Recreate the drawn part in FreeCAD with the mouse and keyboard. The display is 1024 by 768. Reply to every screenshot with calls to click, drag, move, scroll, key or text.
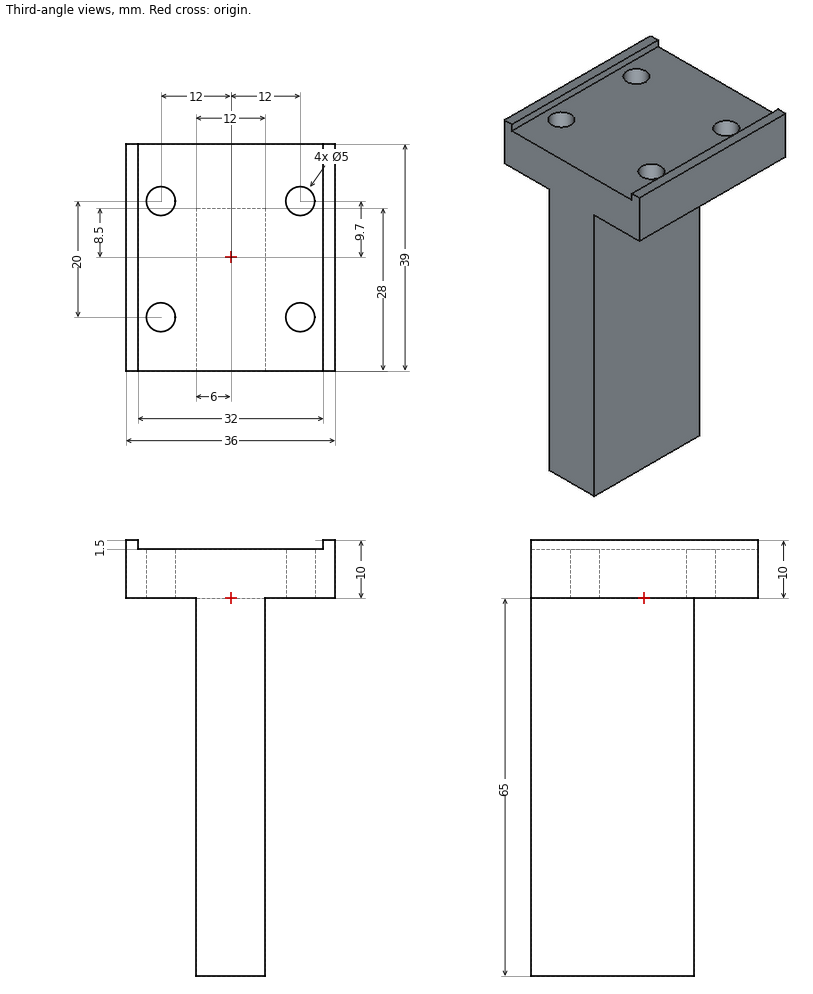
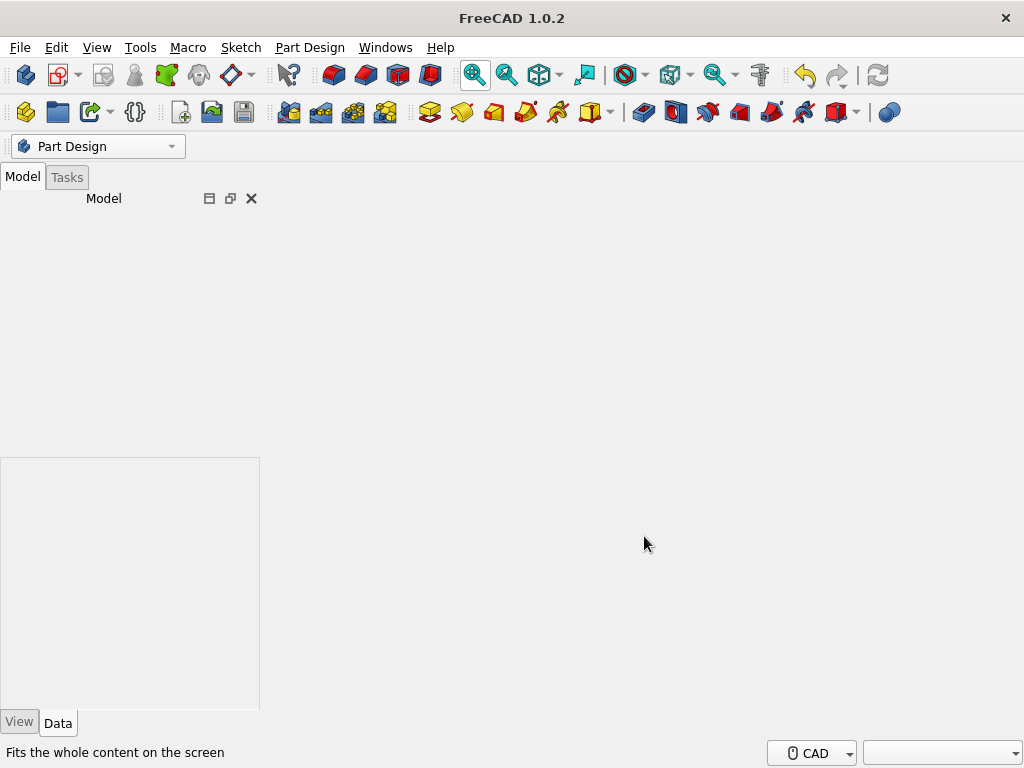
key(ctrl+n)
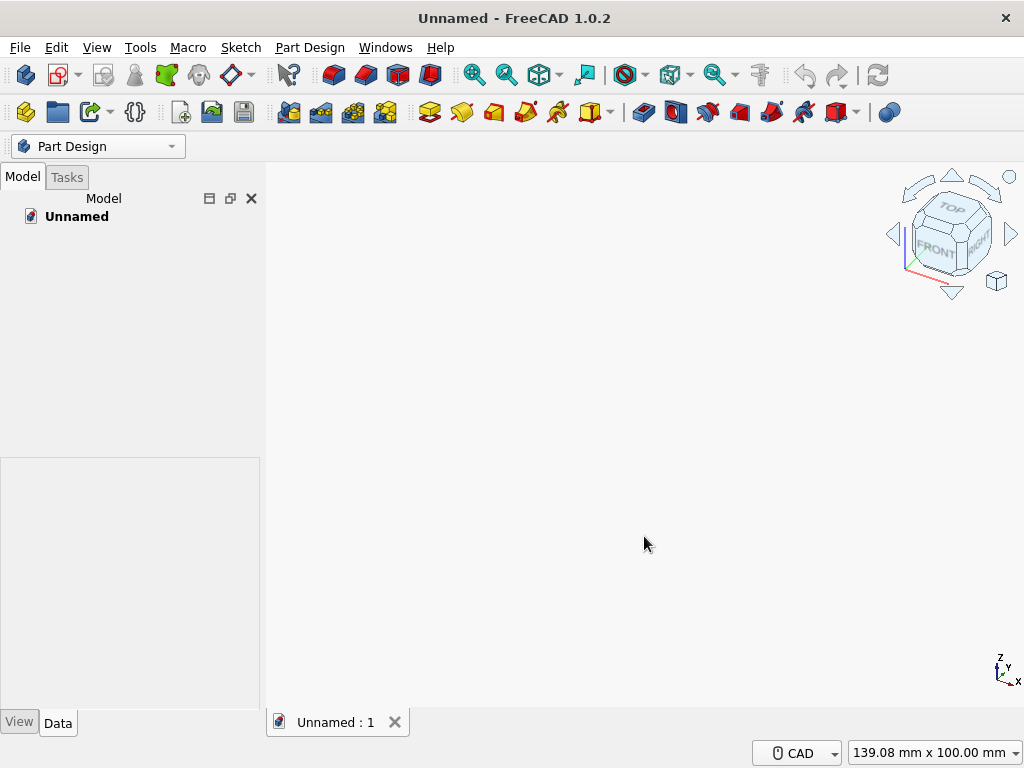
click(58, 76)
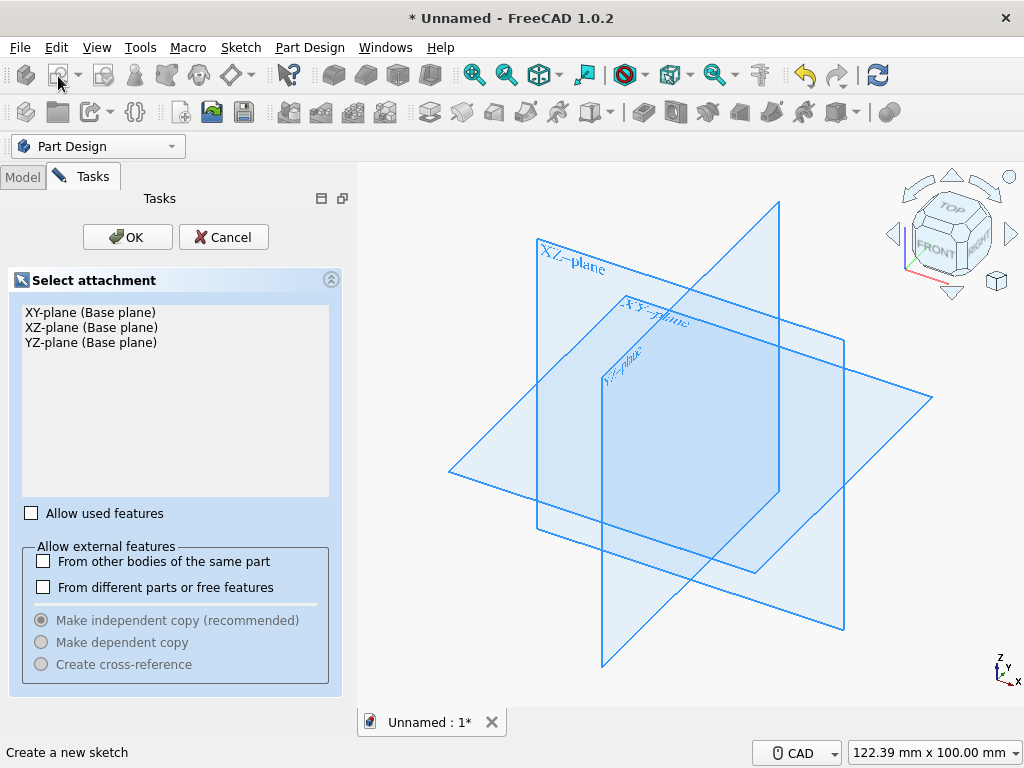
click(82, 312)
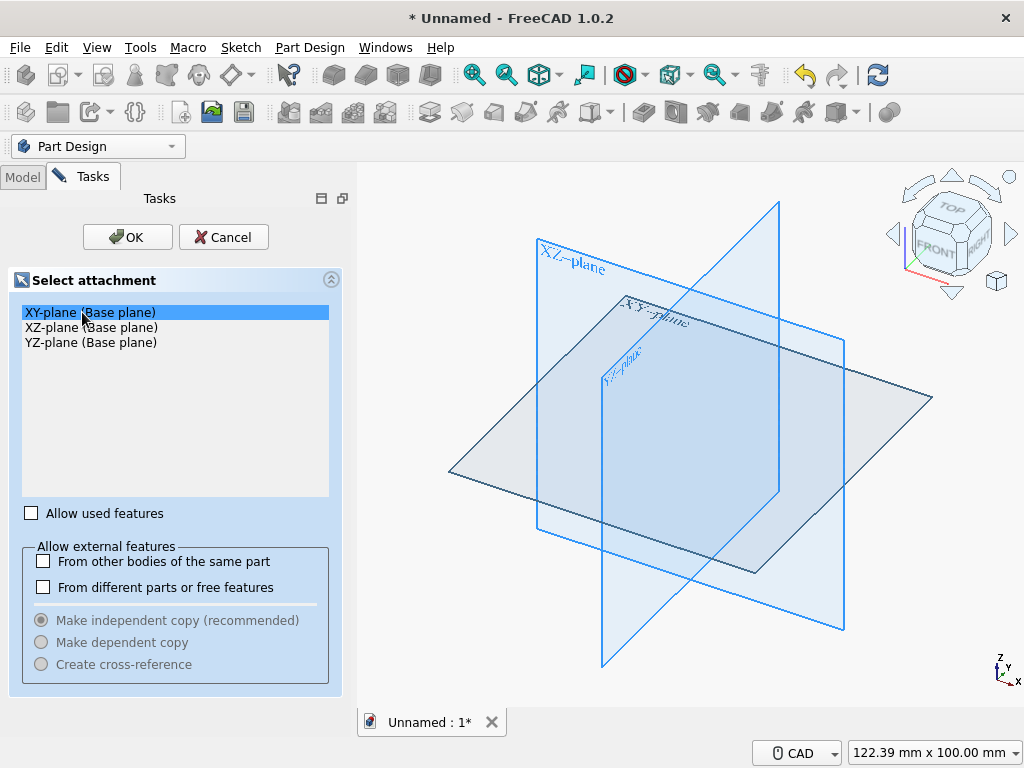
click(128, 237)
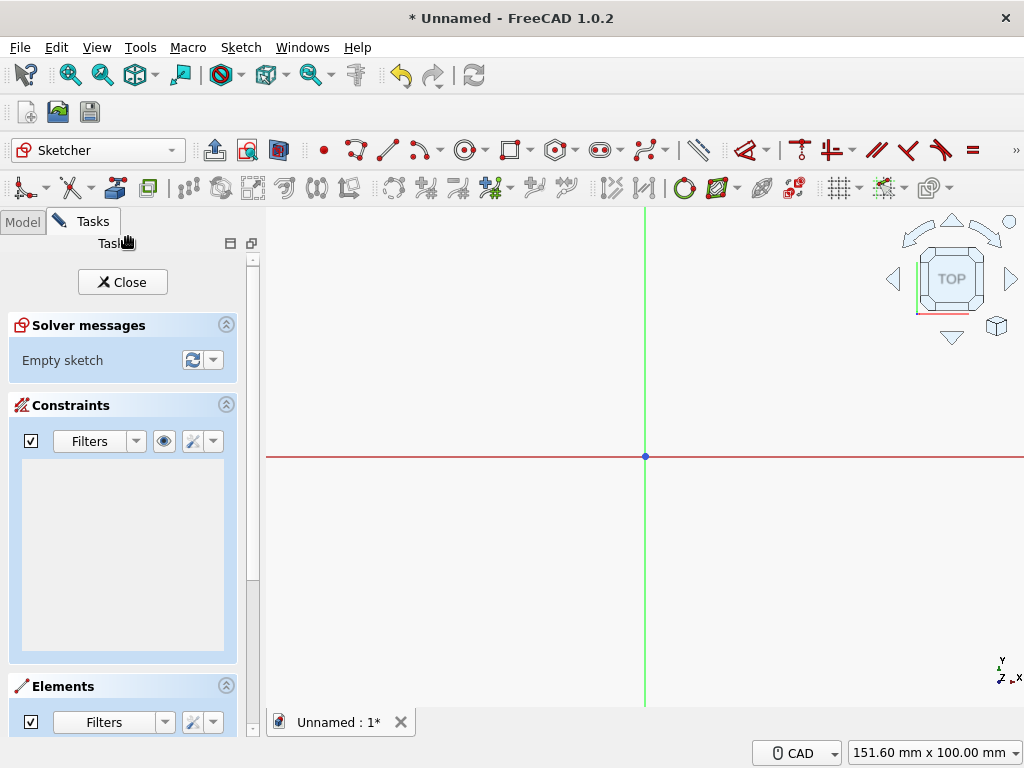
scroll(784, 457, up, 2)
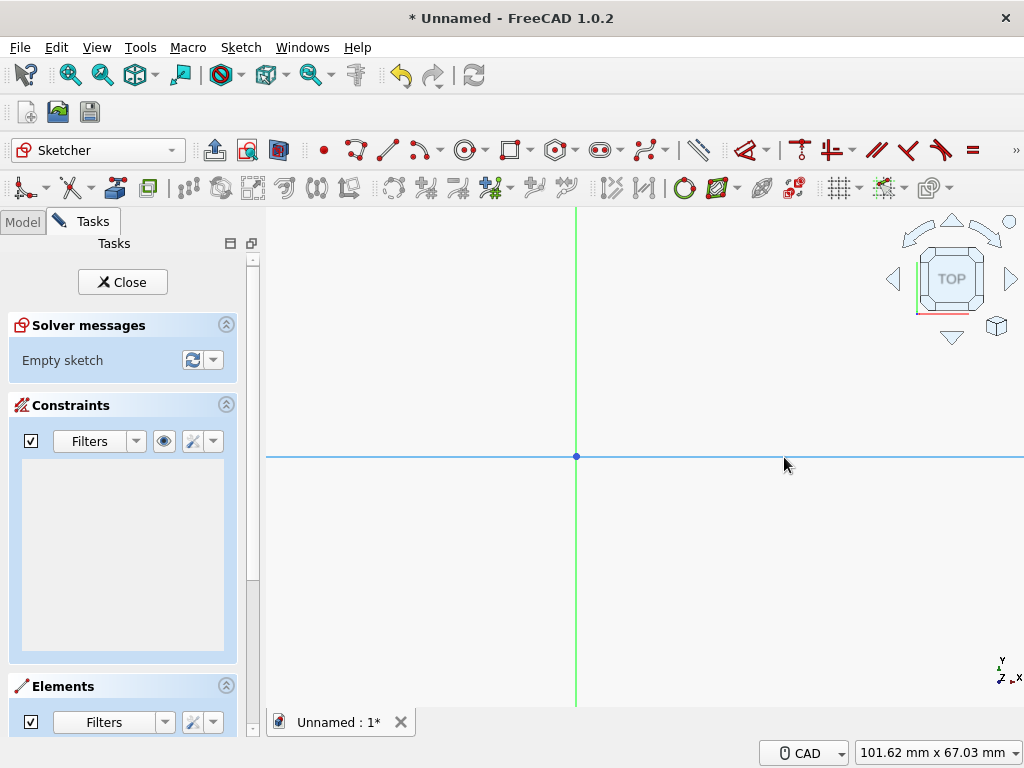
key(g)
key(v)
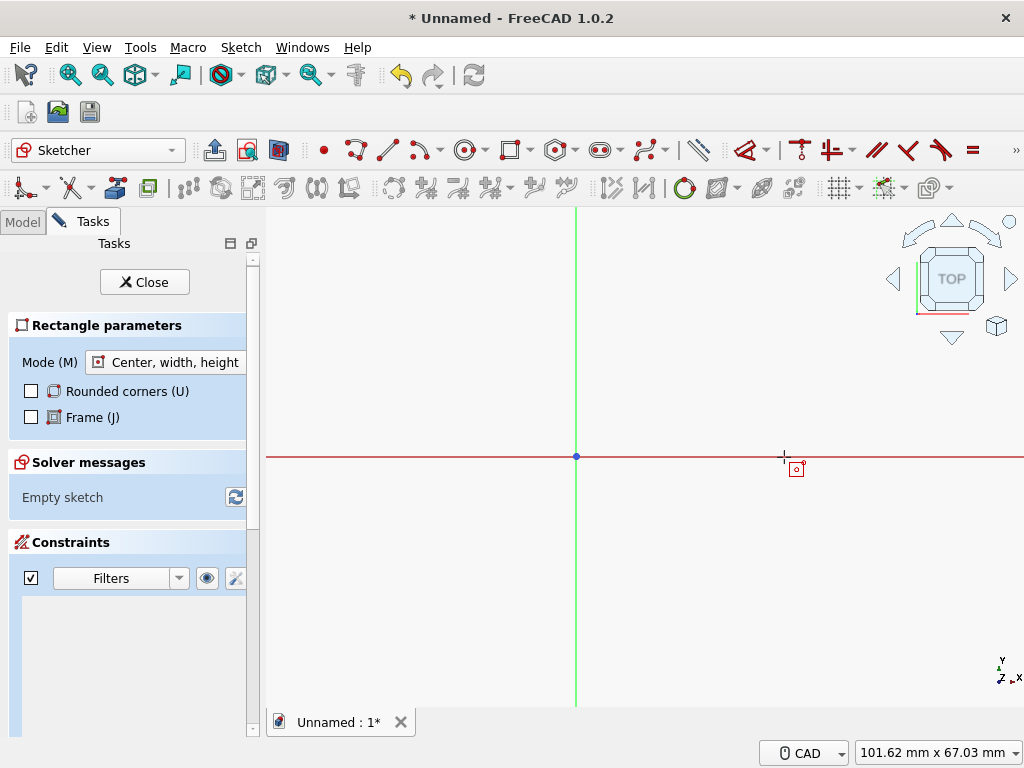
click(576, 457)
move(711, 311)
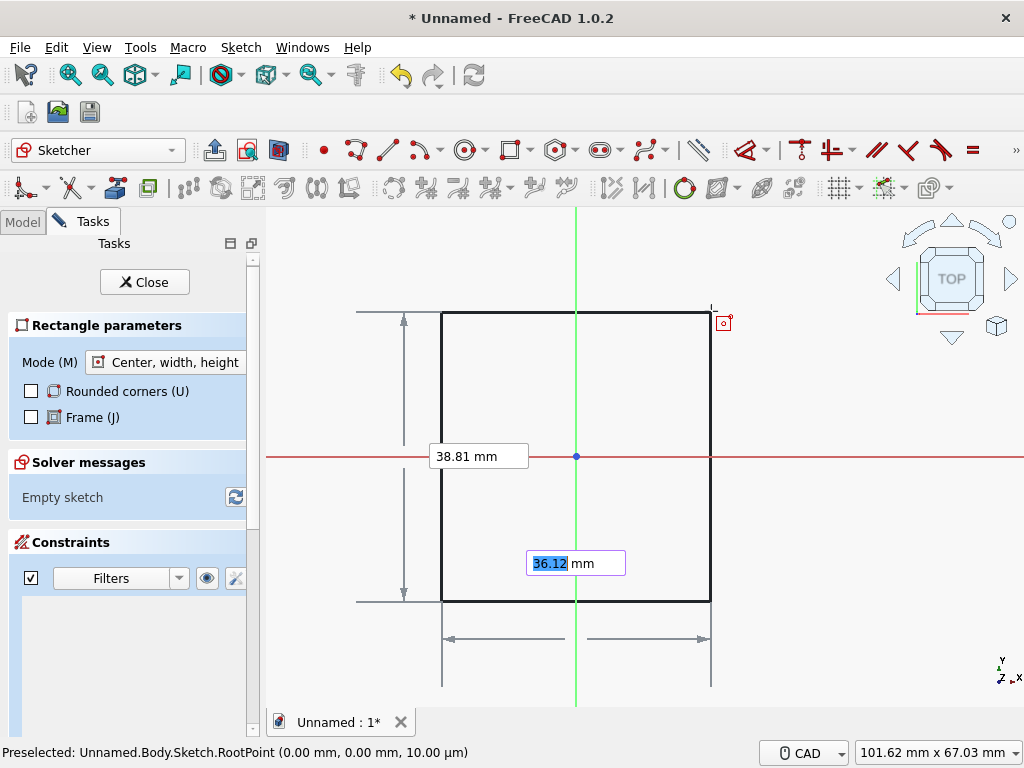
text(36)
key(Tab)
text(39)
key(Return)
key(Escape)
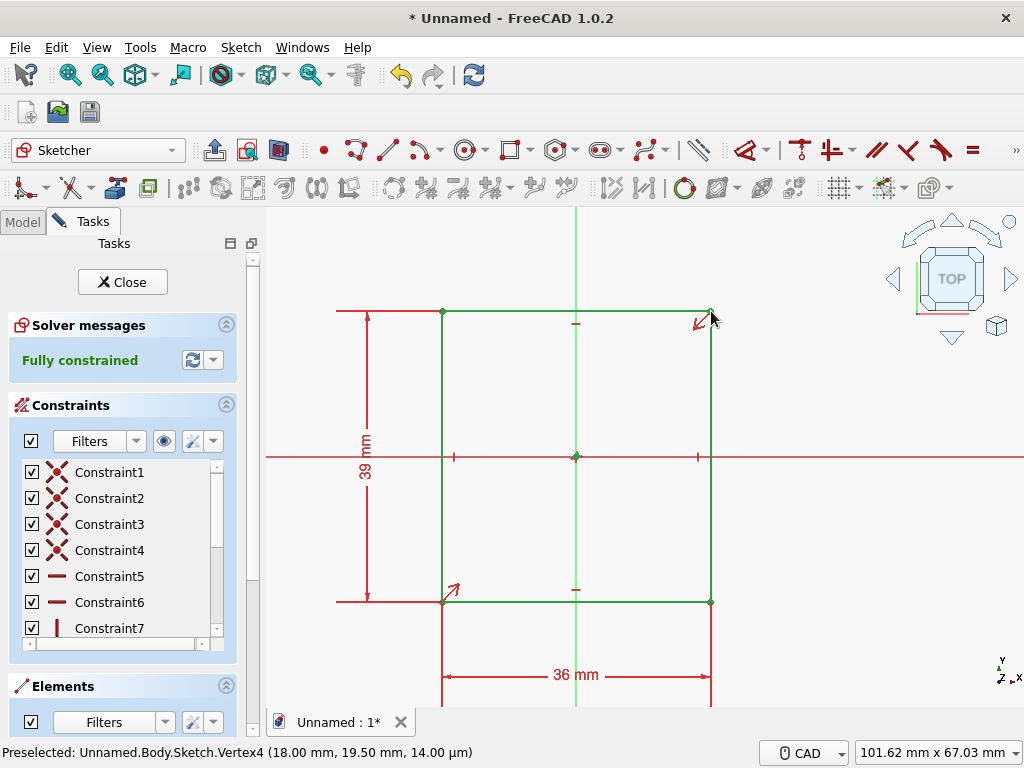
click(123, 282)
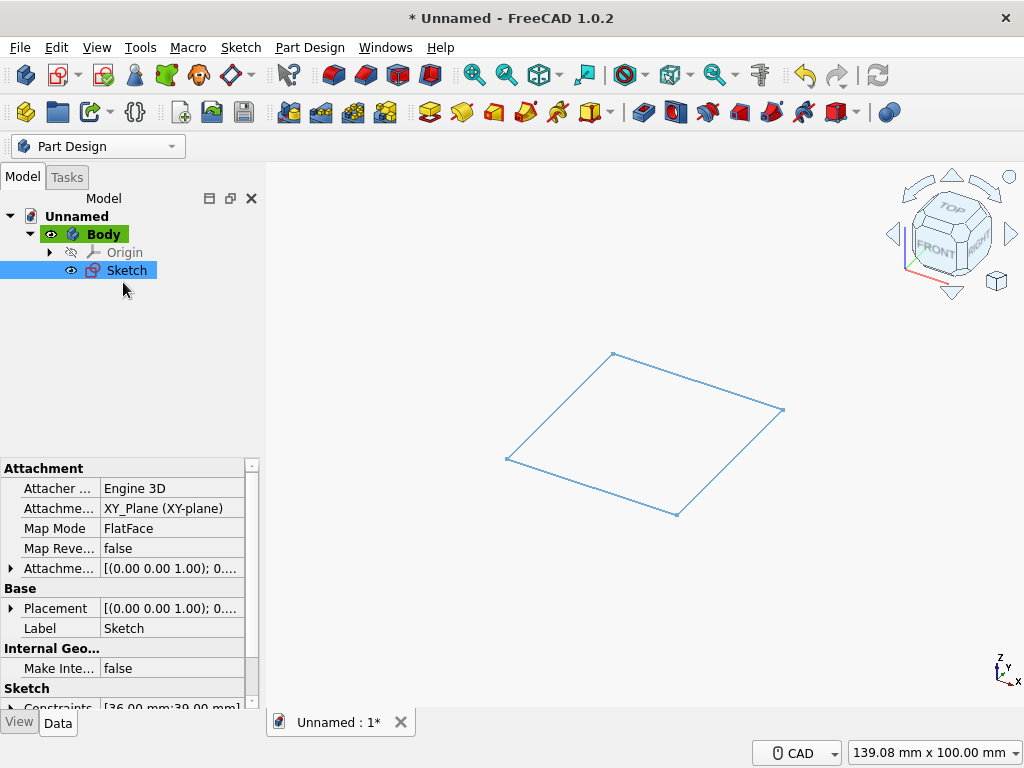
click(430, 112)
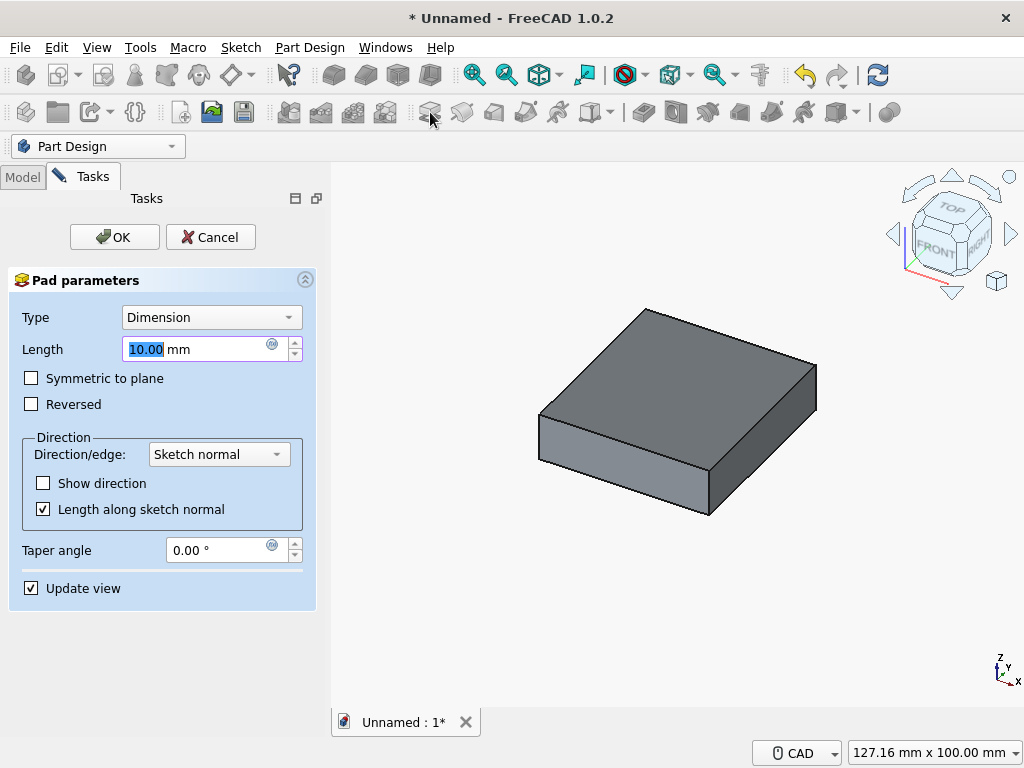
text(10)
key(Tab)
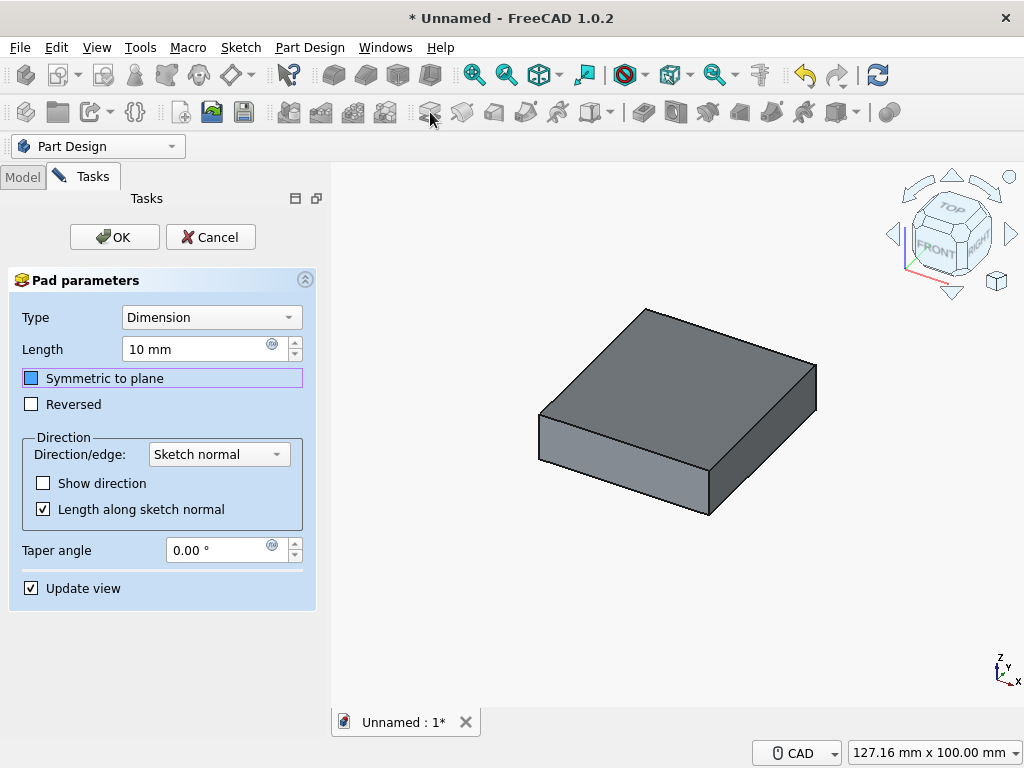
click(115, 237)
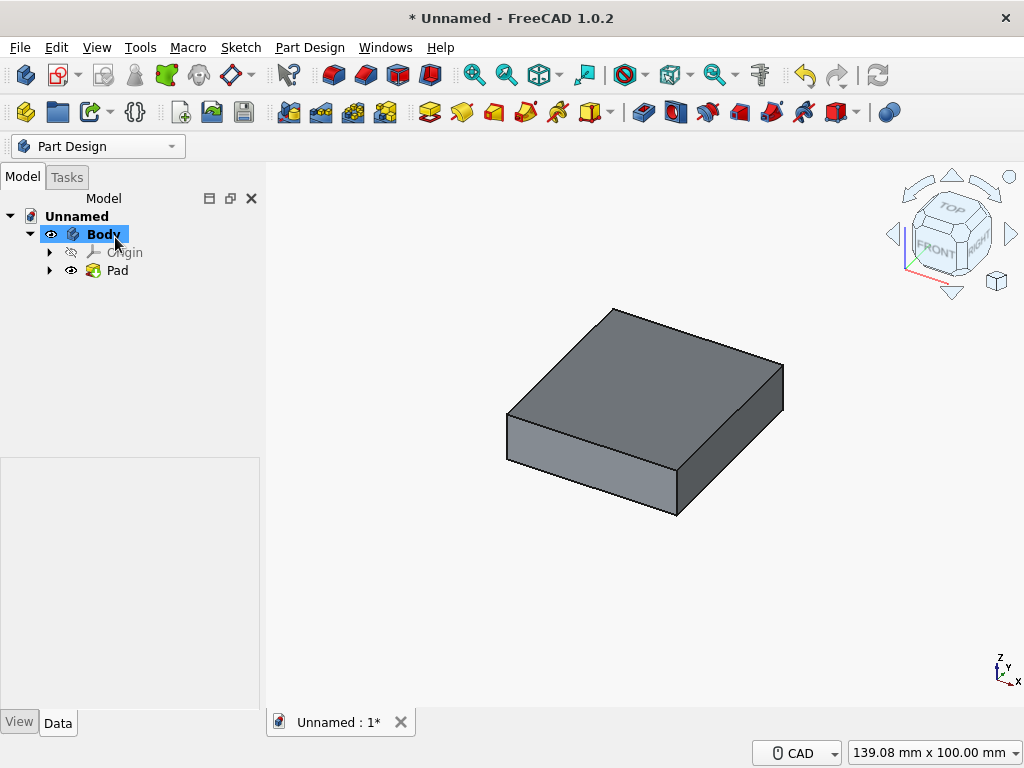
key(v)
key(f)